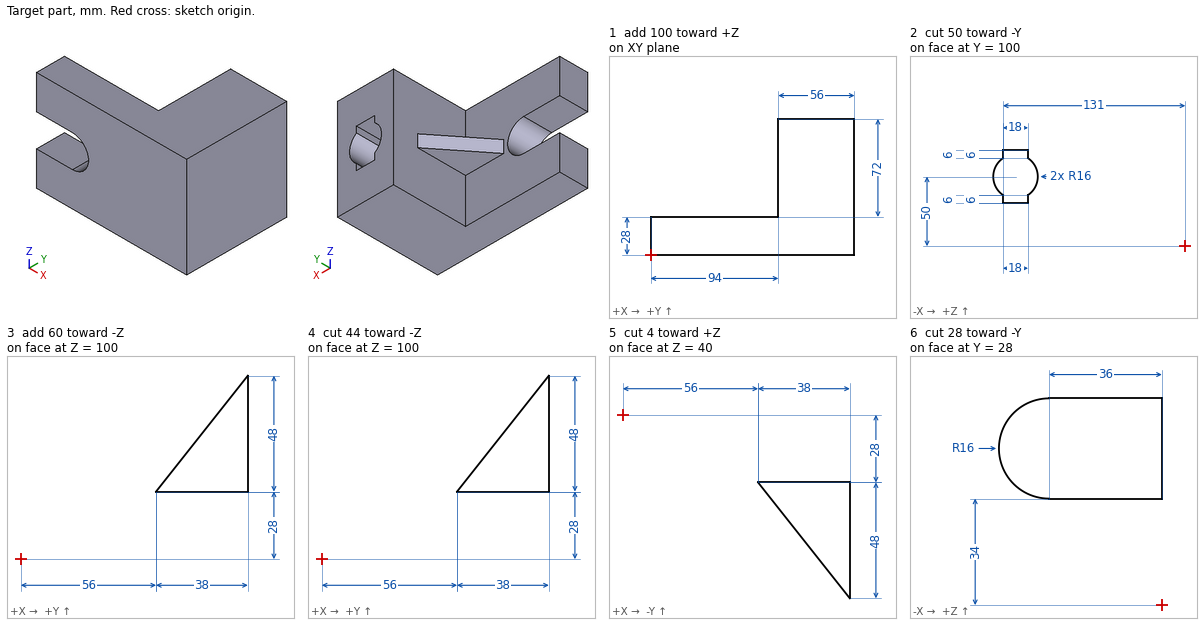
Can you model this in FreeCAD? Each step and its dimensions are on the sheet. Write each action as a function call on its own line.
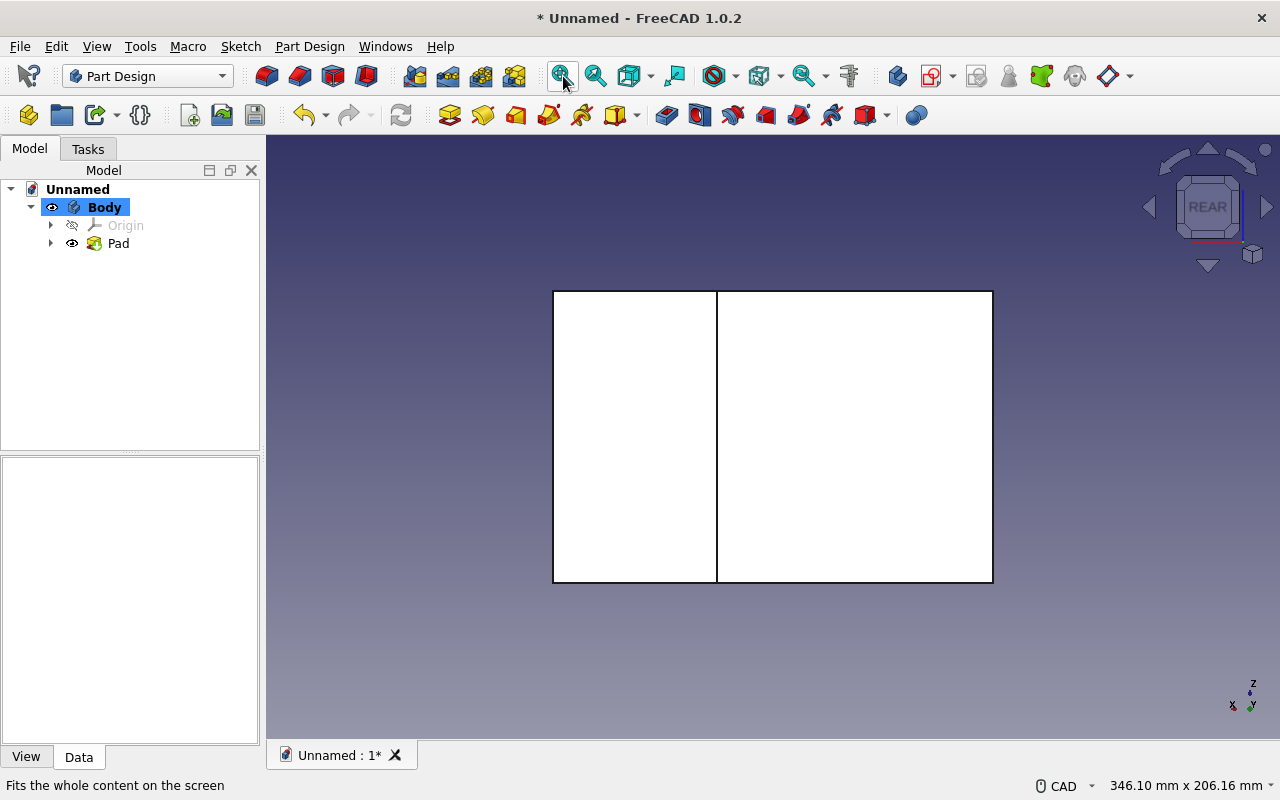
click(635, 394)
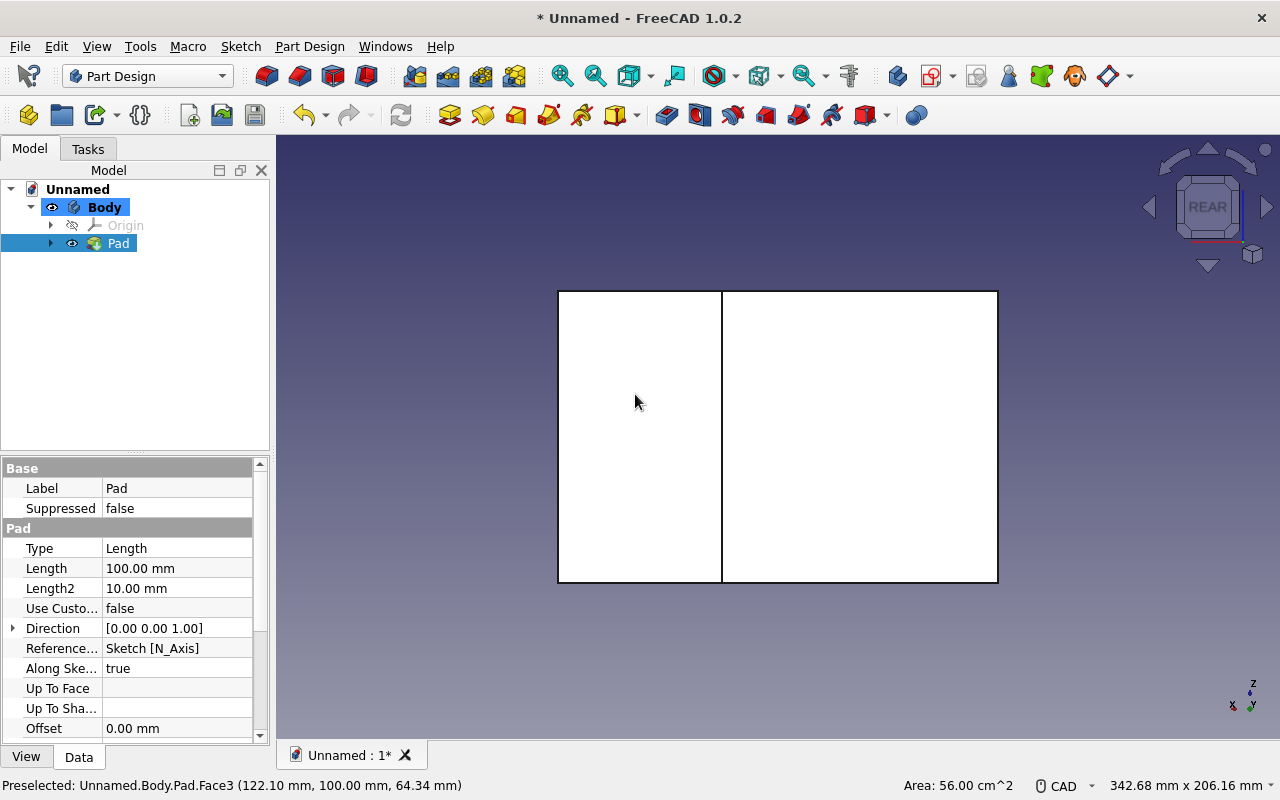
click(930, 76)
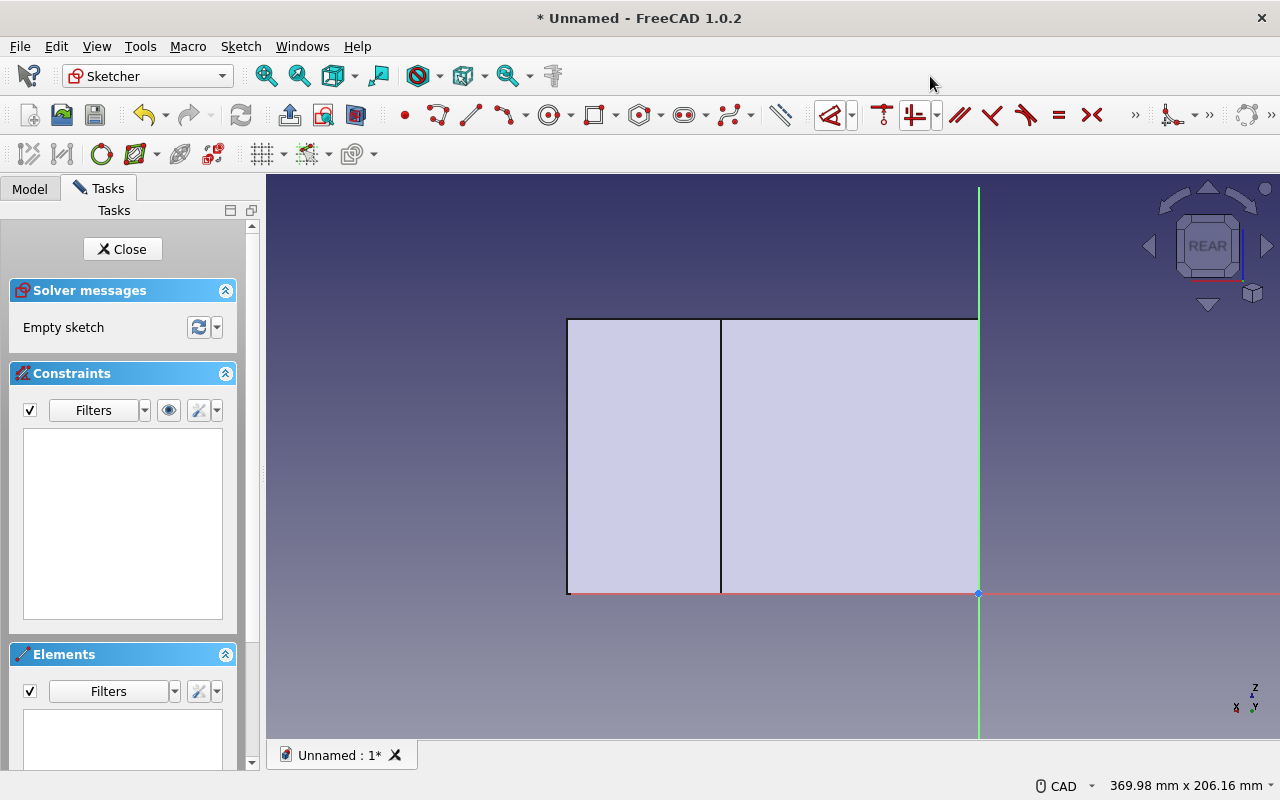
scroll(618, 456, up, 6)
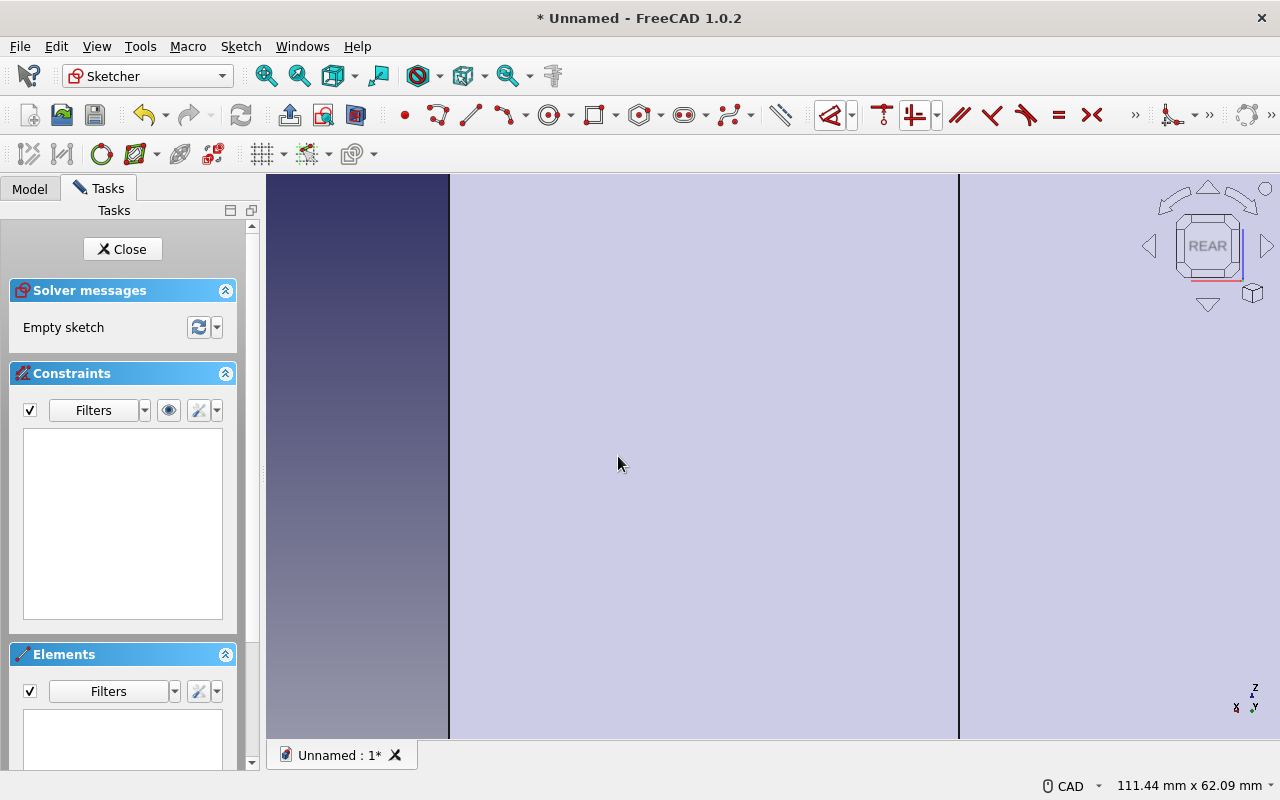
click(438, 116)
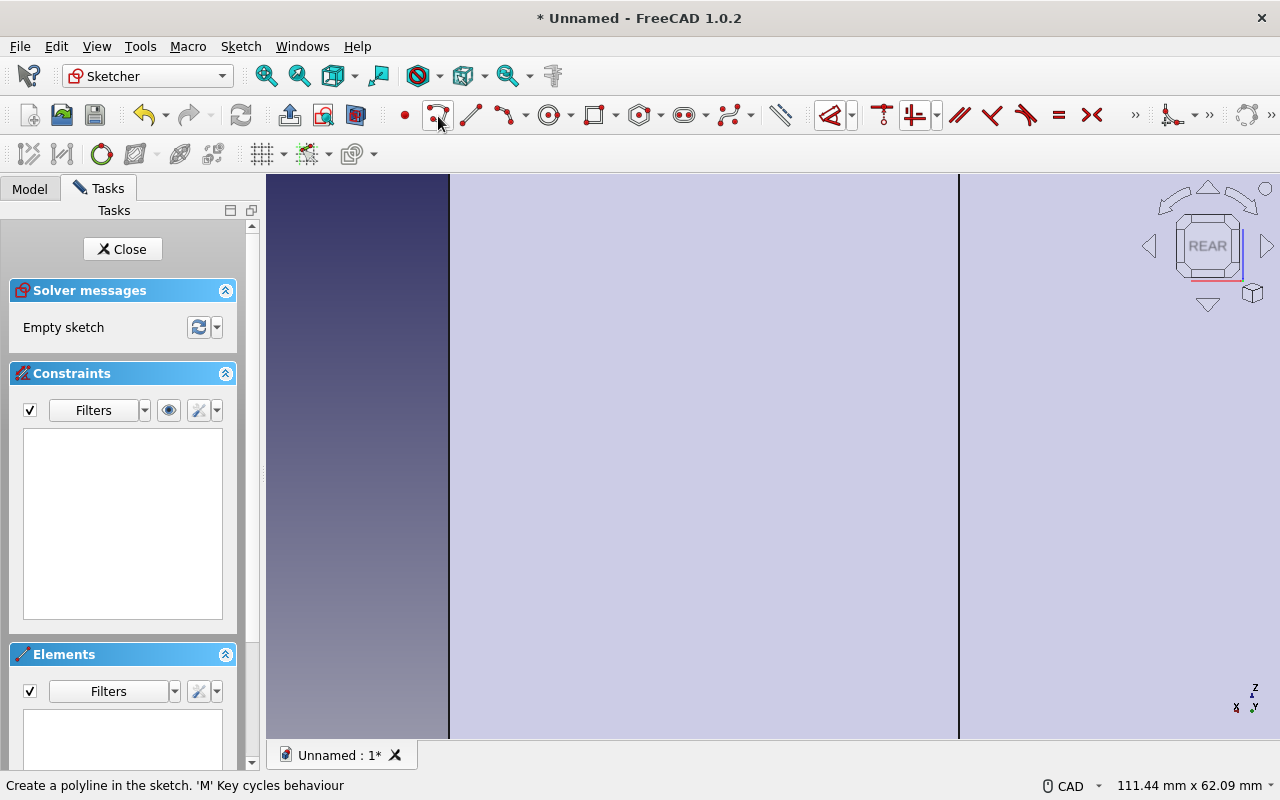
click(622, 577)
click(622, 631)
click(786, 631)
click(786, 577)
right_click(786, 577)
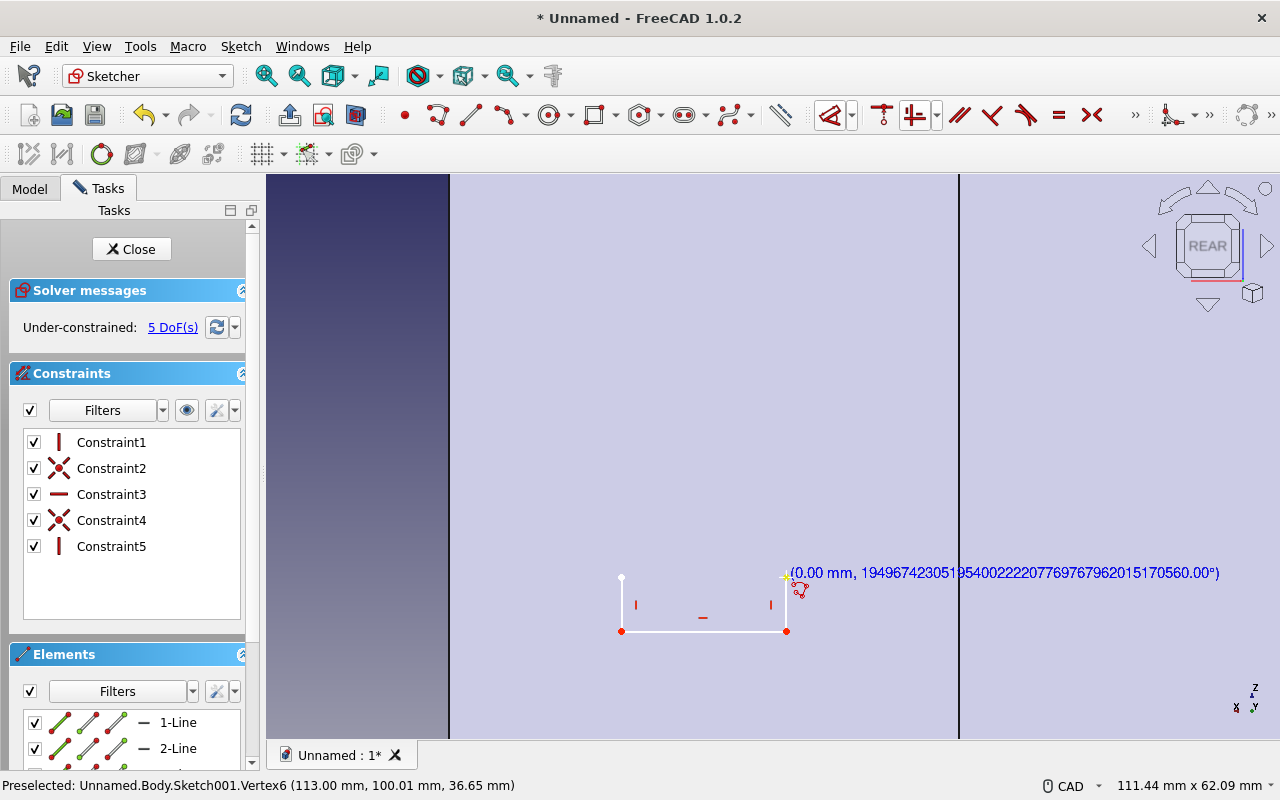
click(786, 336)
click(786, 282)
click(622, 282)
click(622, 336)
right_click(622, 336)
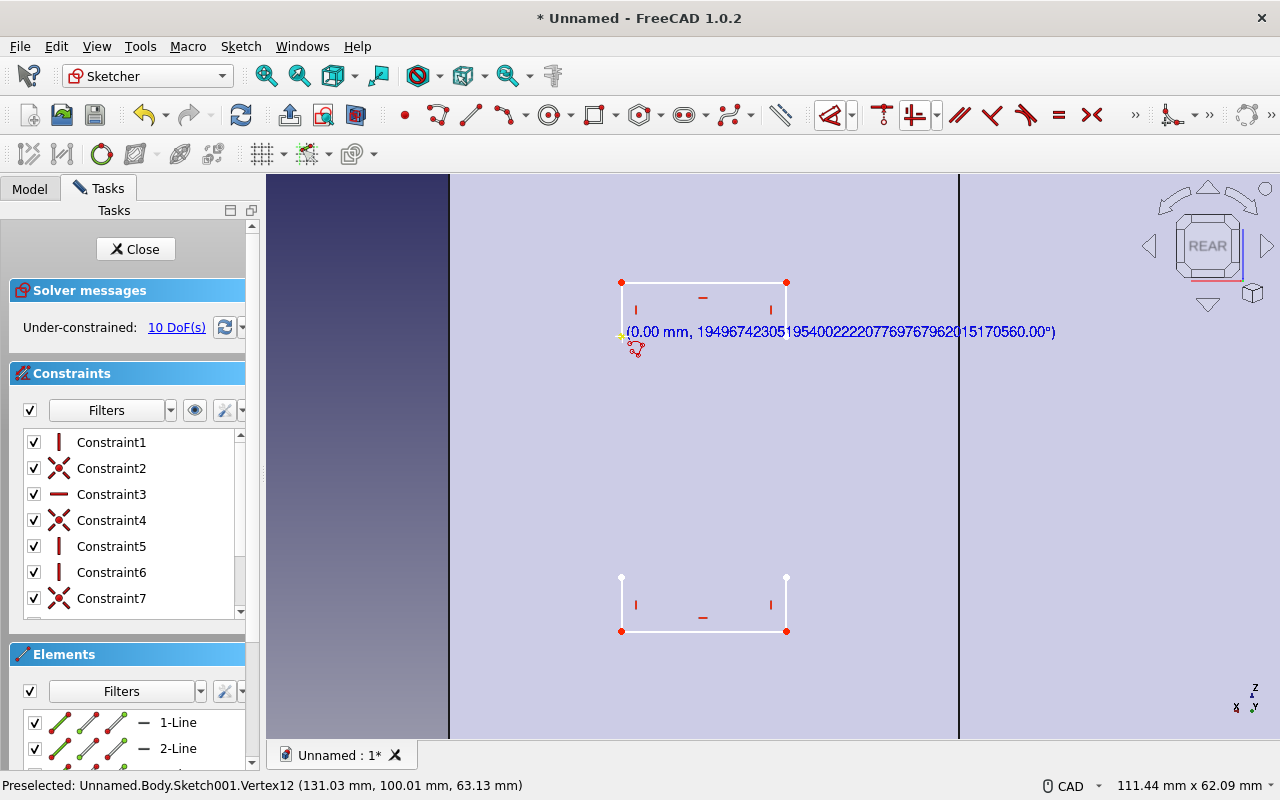
click(504, 116)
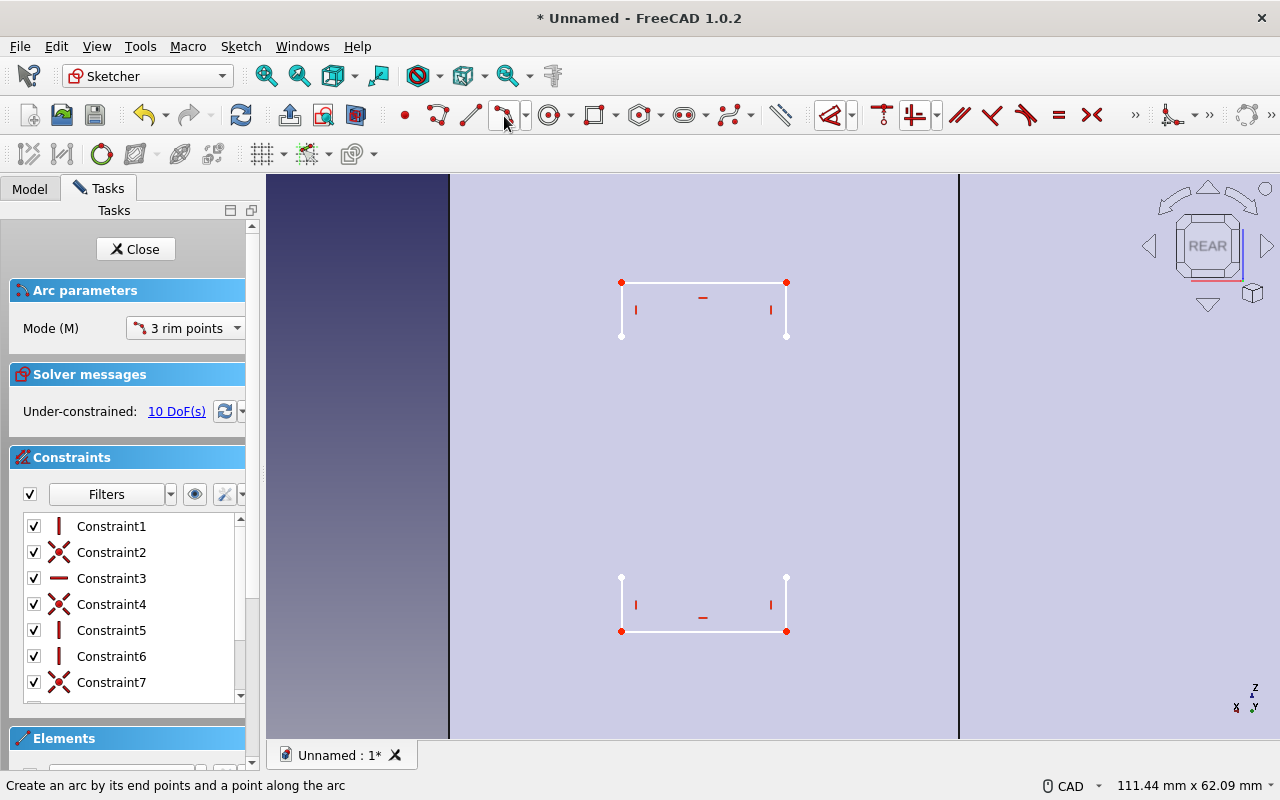
click(786, 578)
click(786, 337)
click(850, 456)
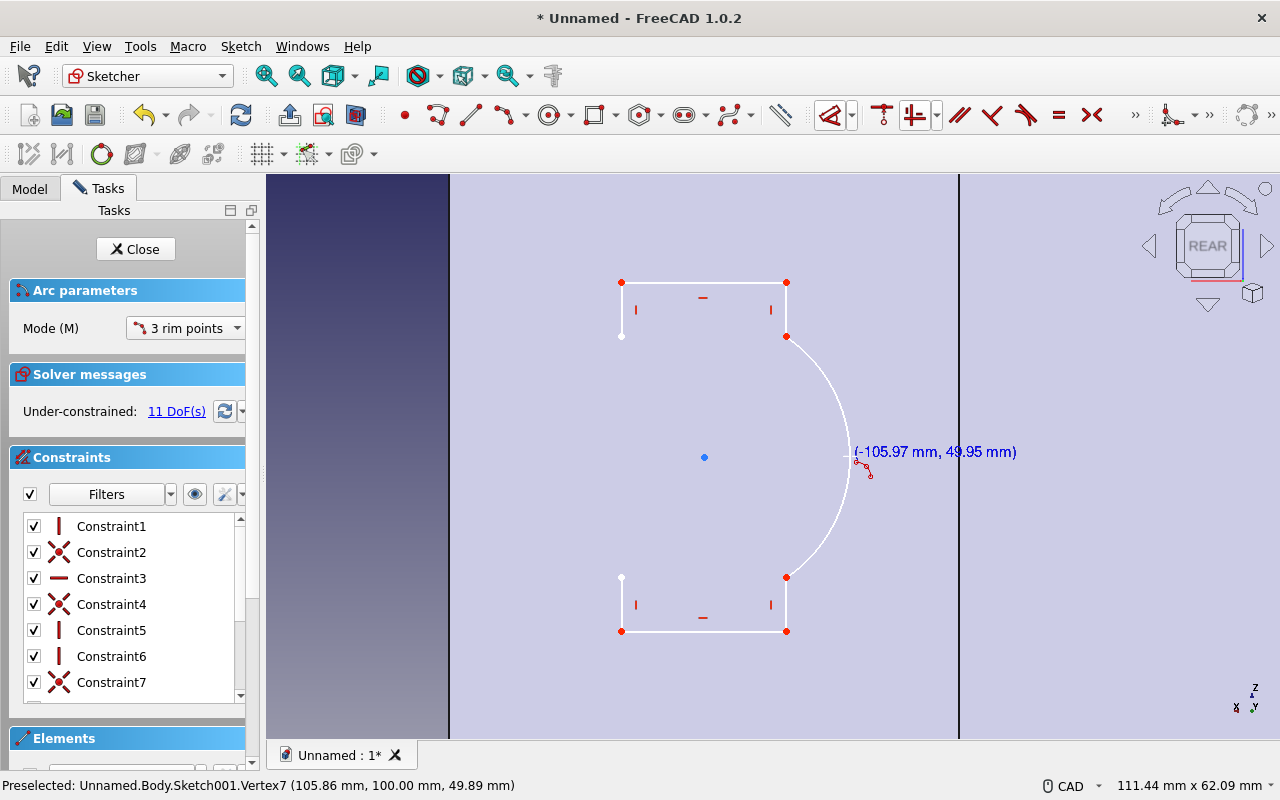
click(622, 337)
click(622, 578)
click(559, 456)
key(Escape)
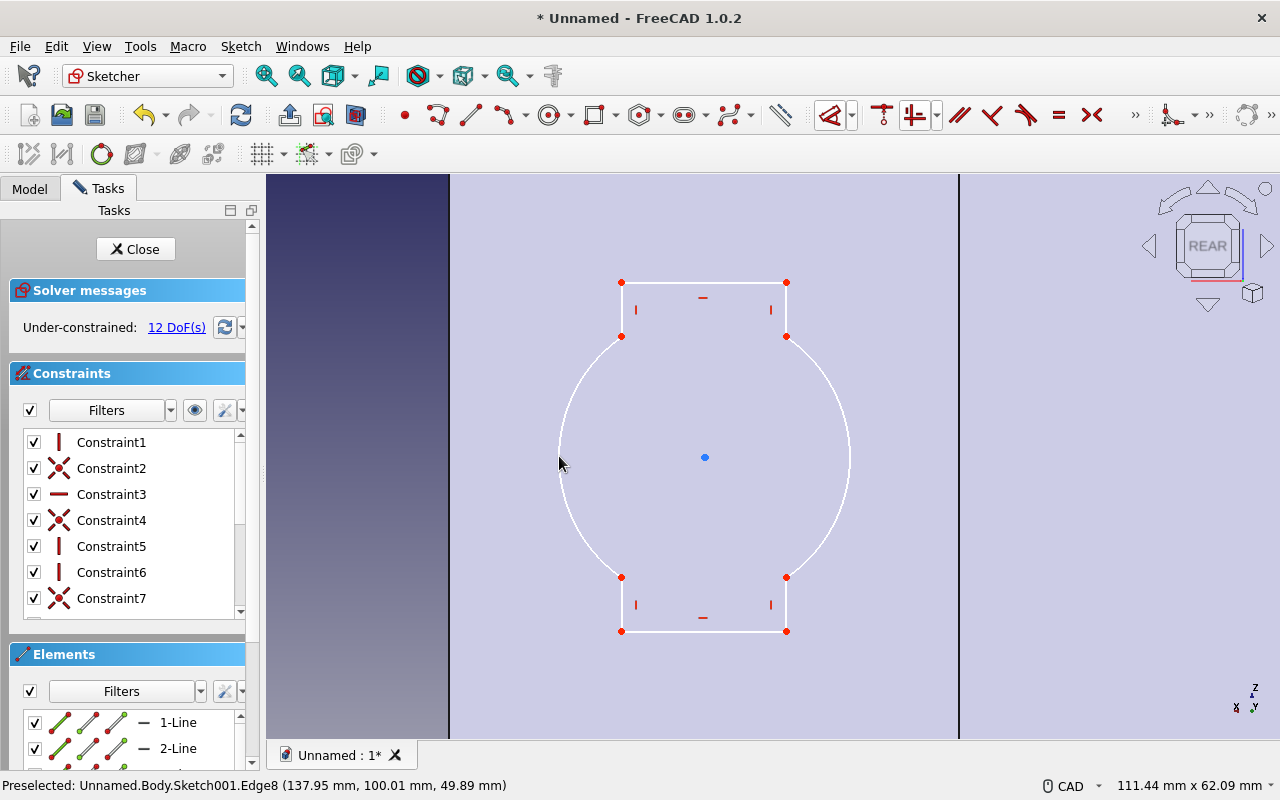
click(839, 513)